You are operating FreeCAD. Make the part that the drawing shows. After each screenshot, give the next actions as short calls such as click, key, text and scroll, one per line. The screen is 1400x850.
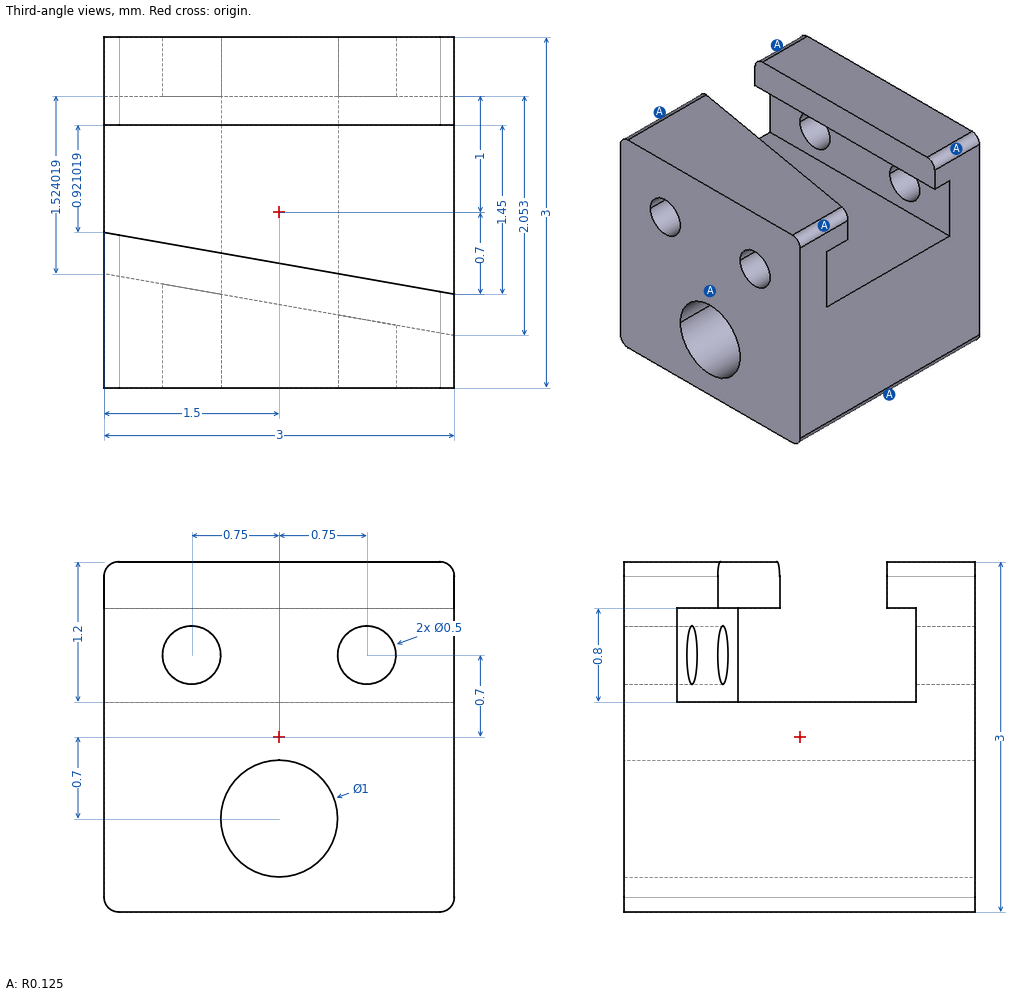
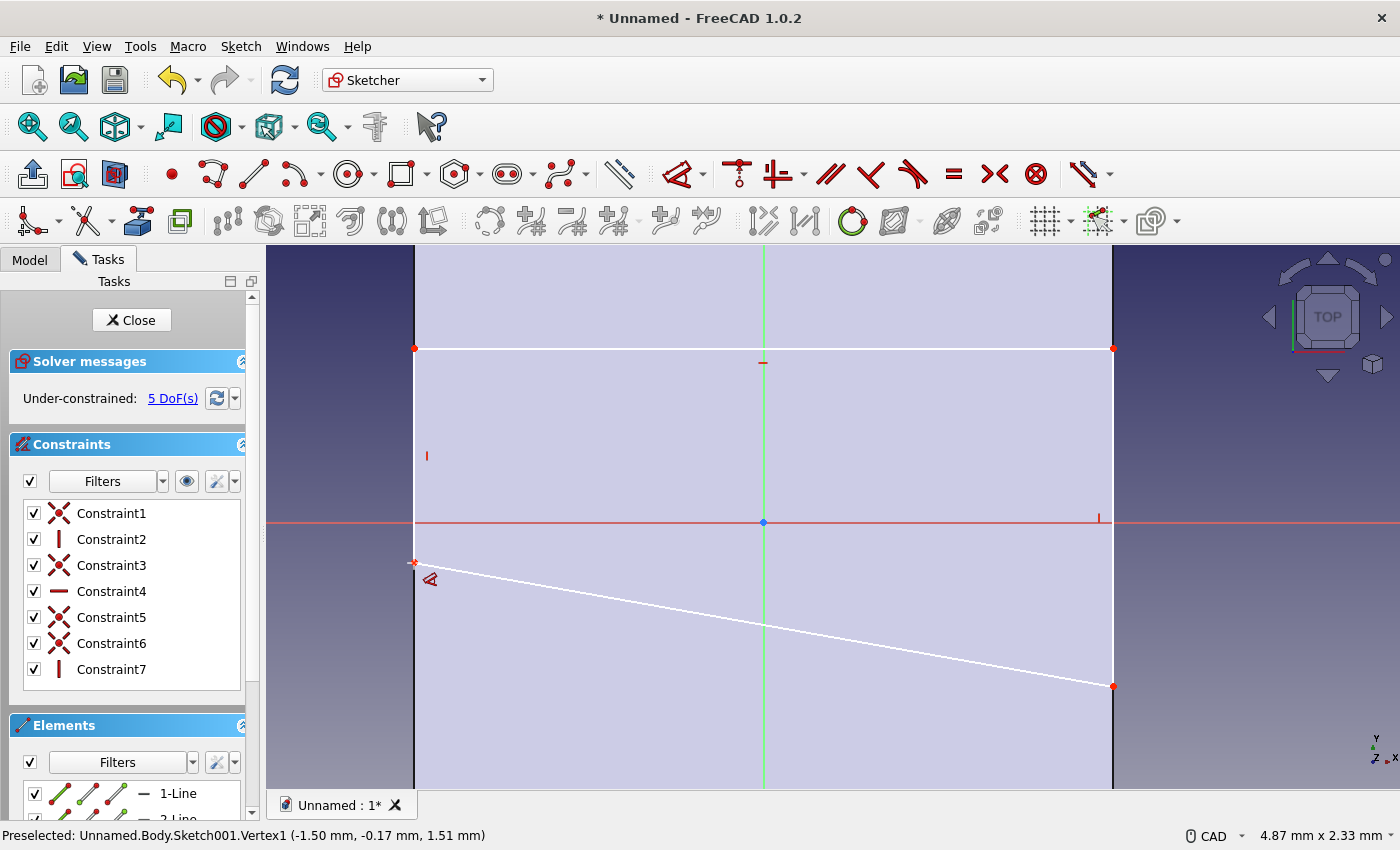
click(903, 349)
click(603, 315)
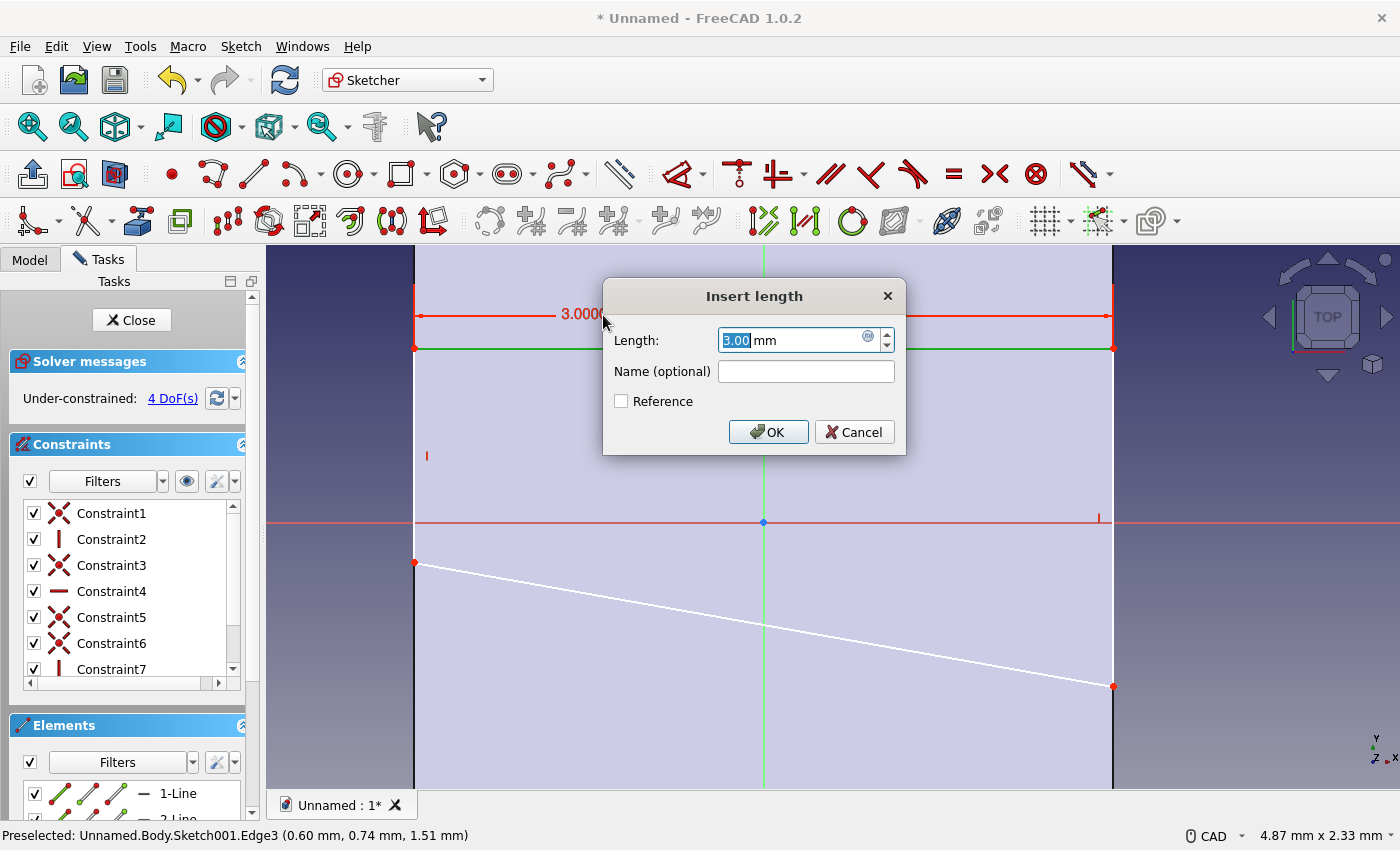
text(3)
key(Return)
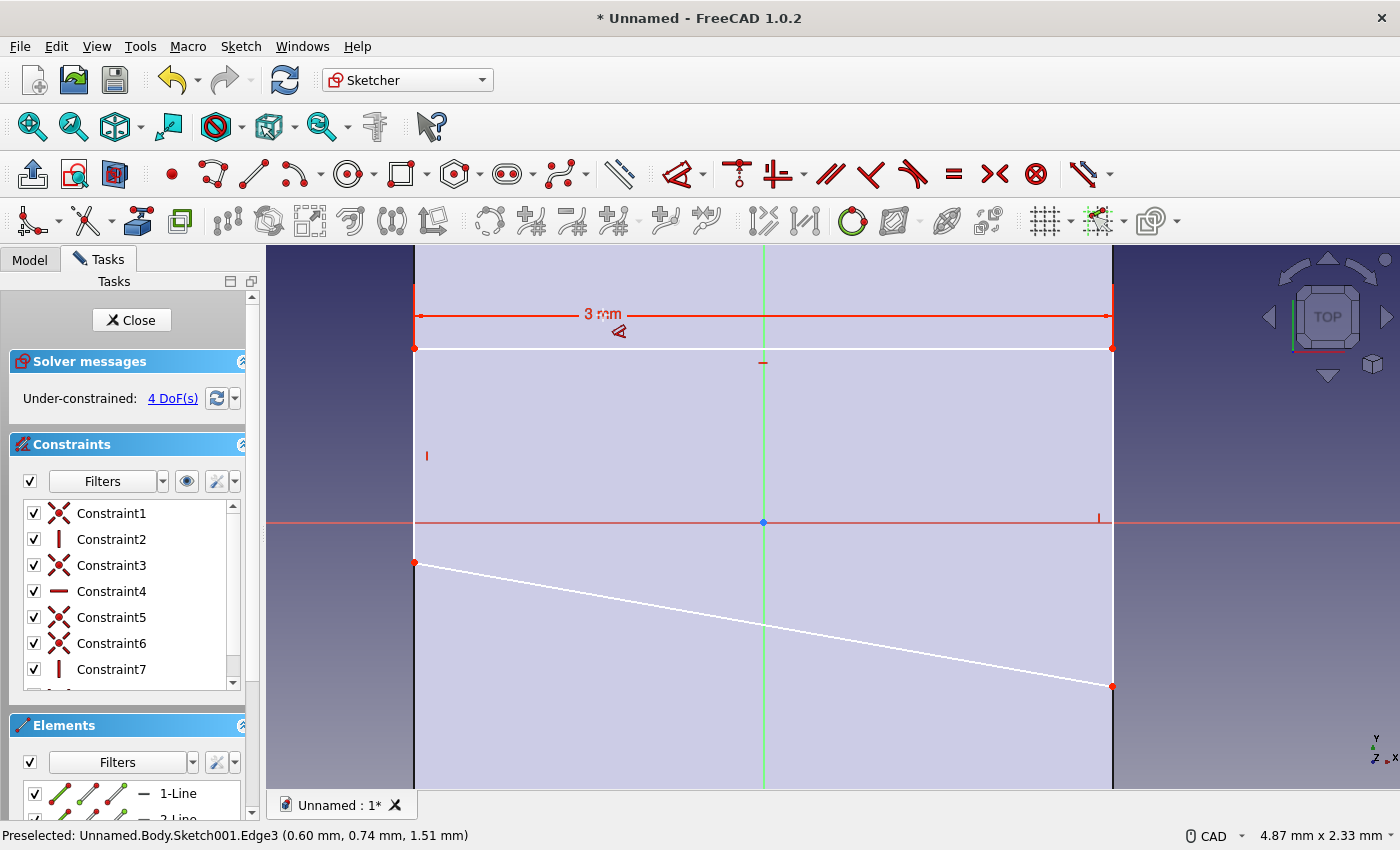
click(1113, 586)
click(1147, 440)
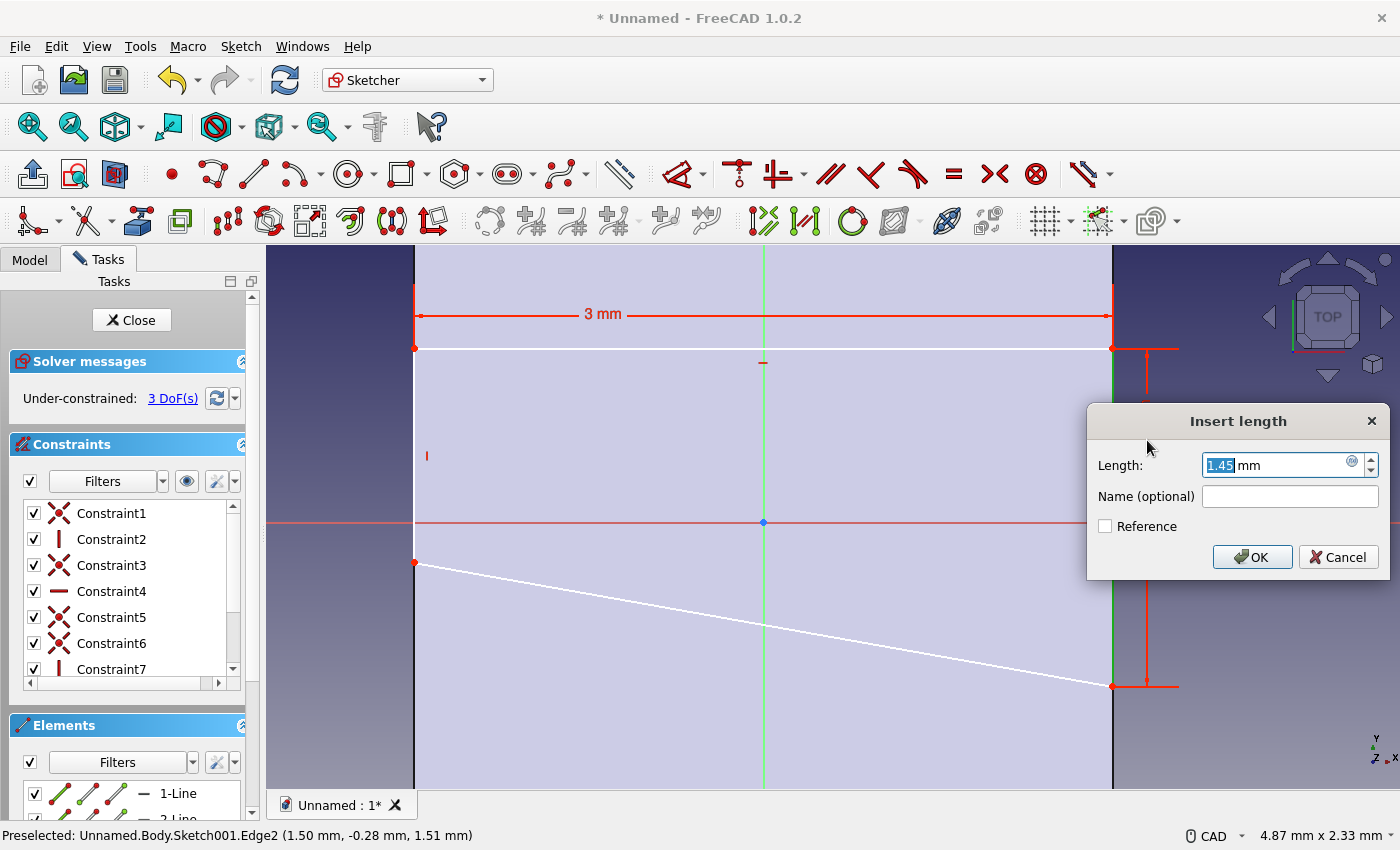
text(1.45)
key(Return)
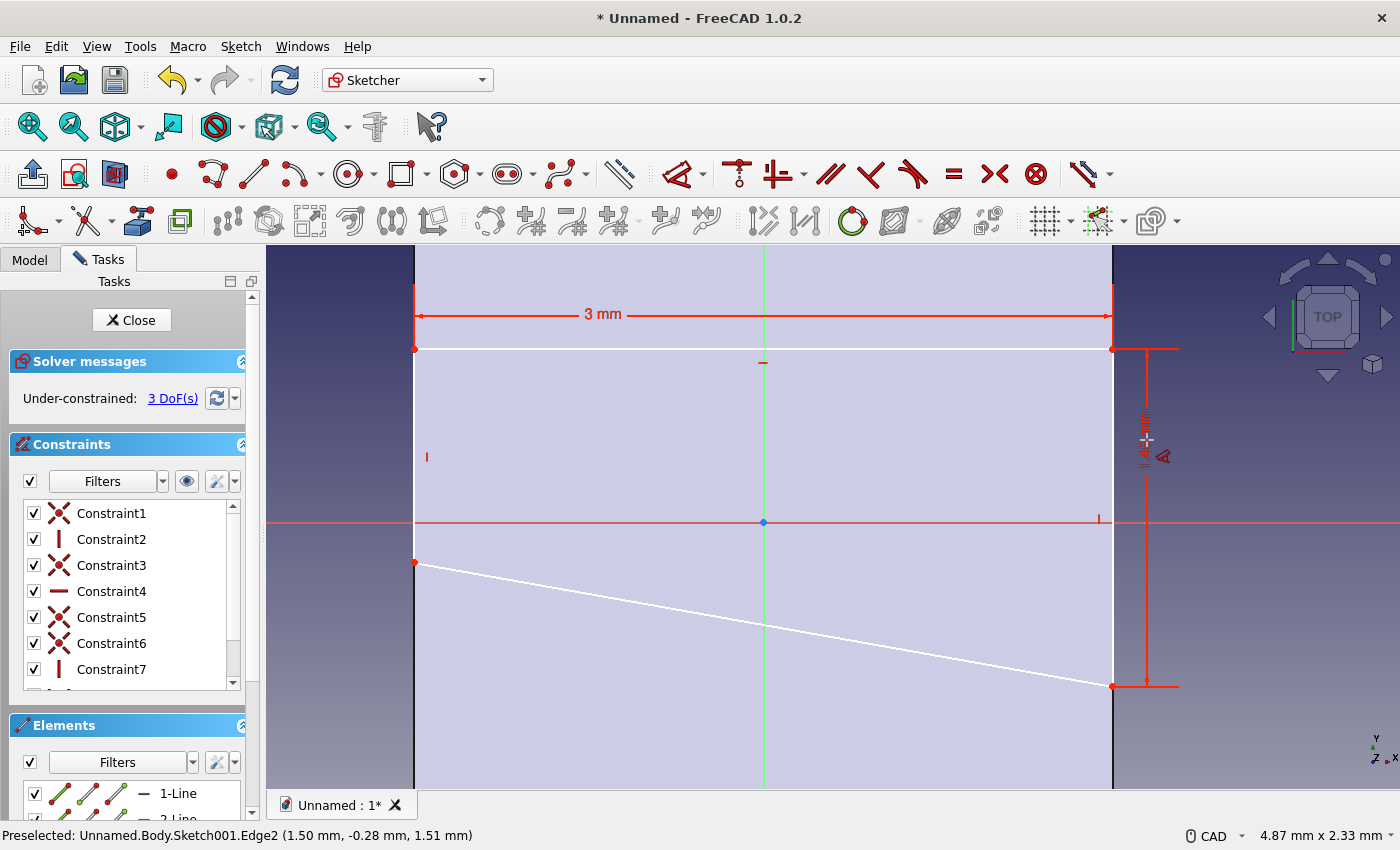
click(414, 563)
click(508, 597)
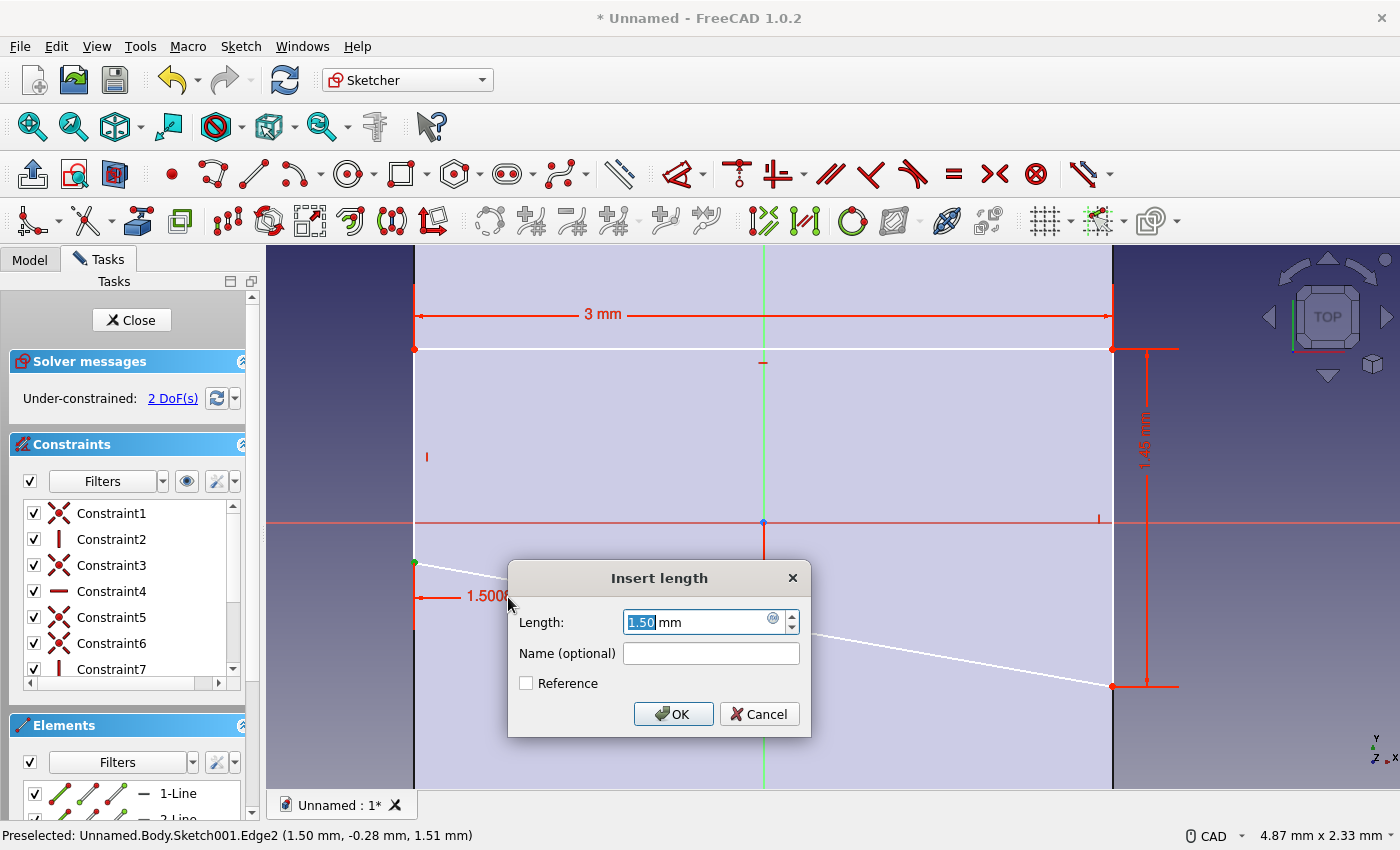
text(1.5)
key(Return)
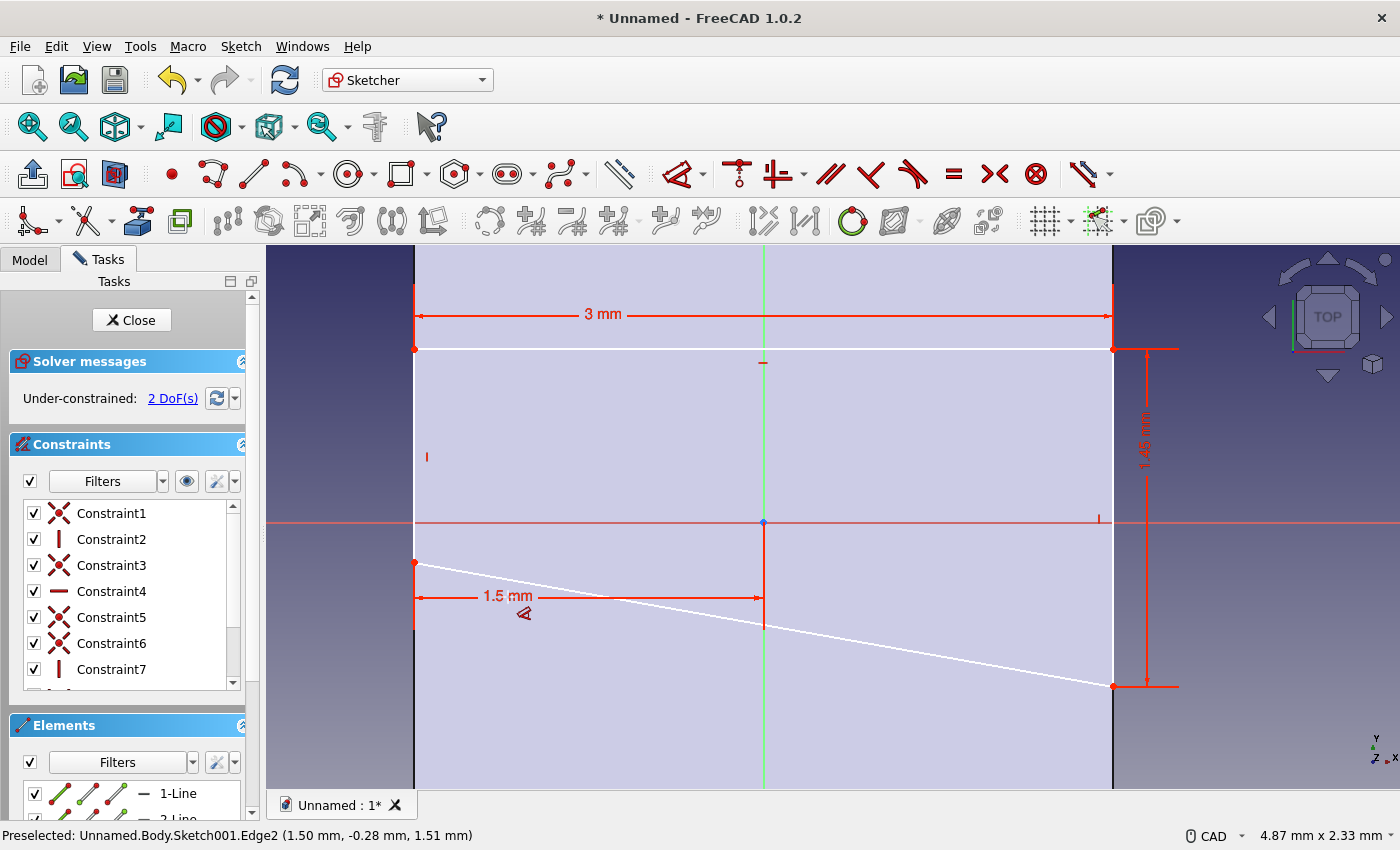
click(1113, 687)
click(1147, 605)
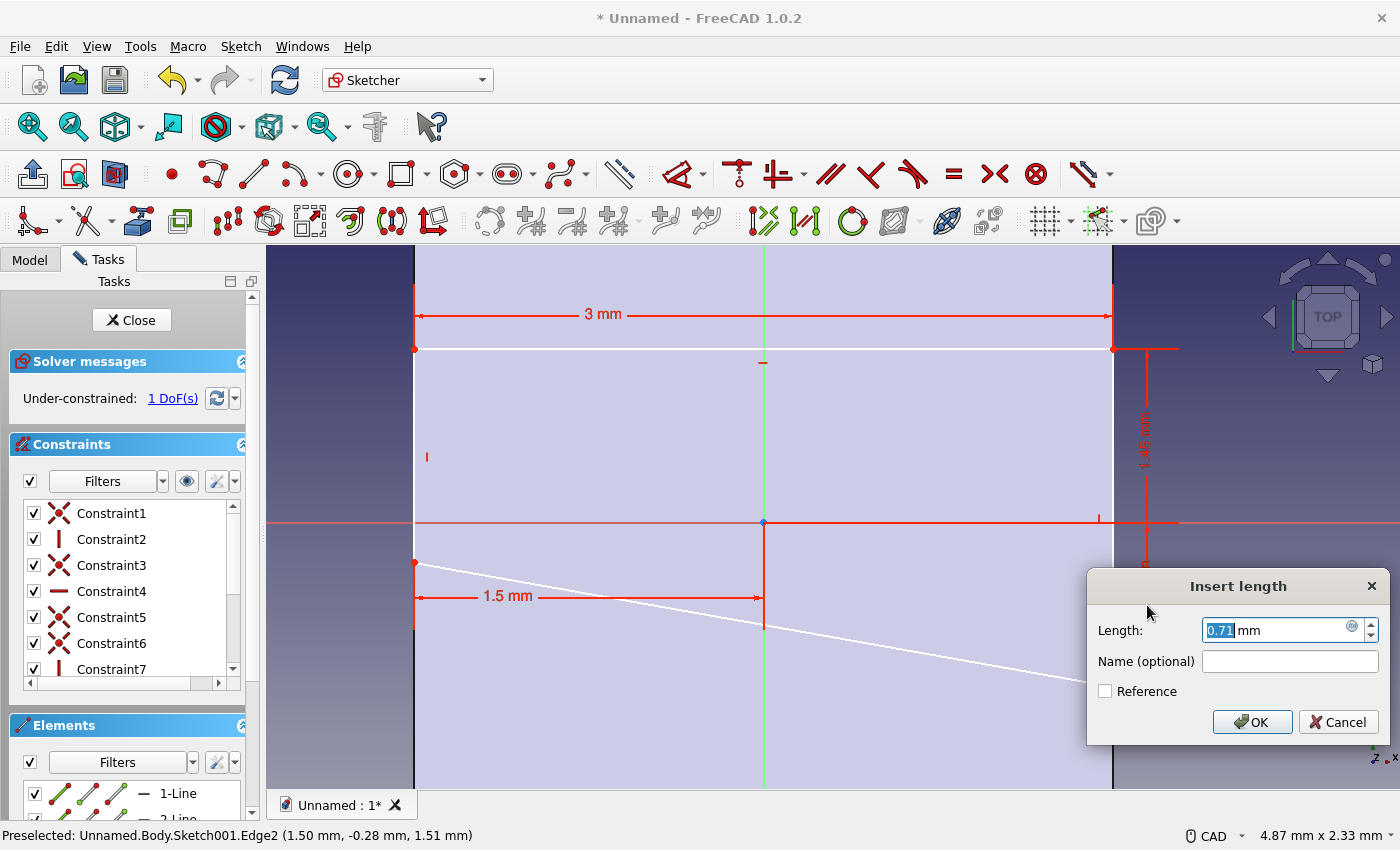
text(0.7)
key(Return)